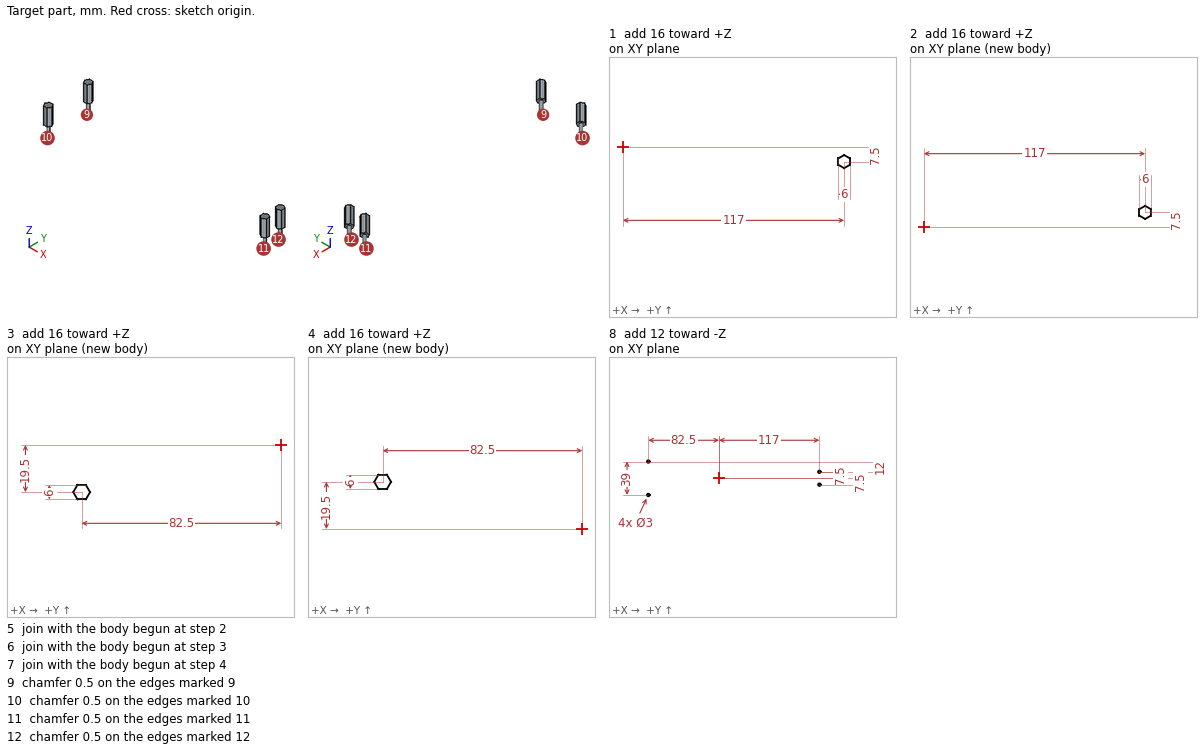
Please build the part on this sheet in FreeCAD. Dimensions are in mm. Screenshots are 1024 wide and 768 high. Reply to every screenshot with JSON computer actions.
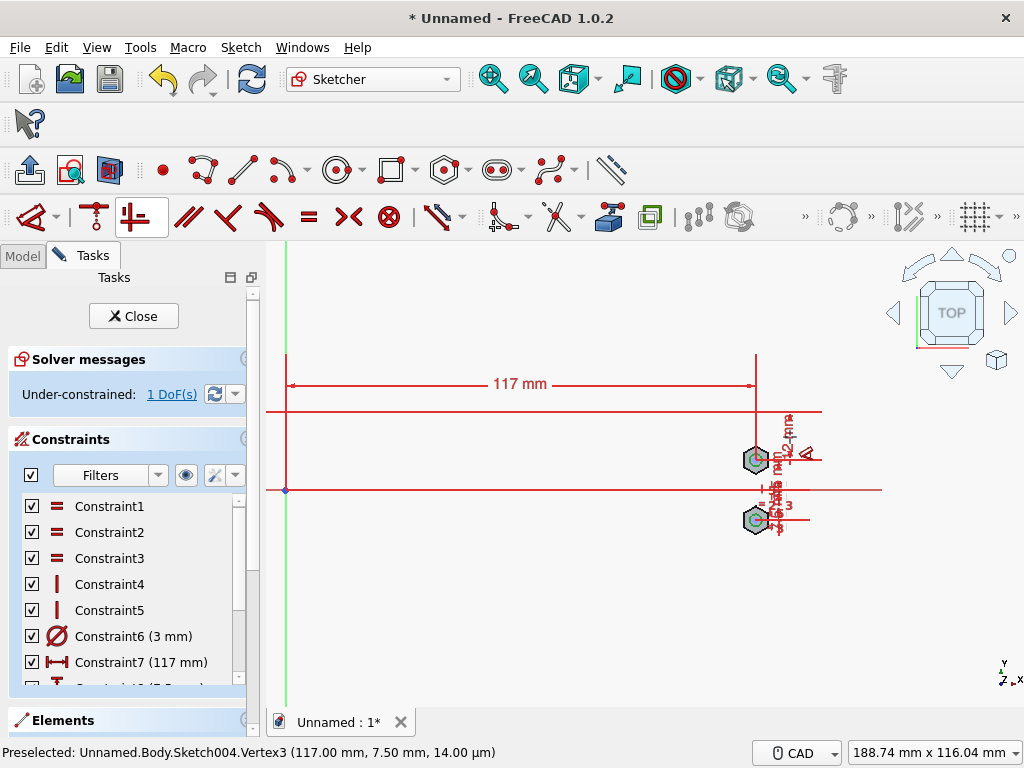
{"action": "scroll", "coordinate": [757, 461], "scroll_direction": "down", "scroll_amount": 4}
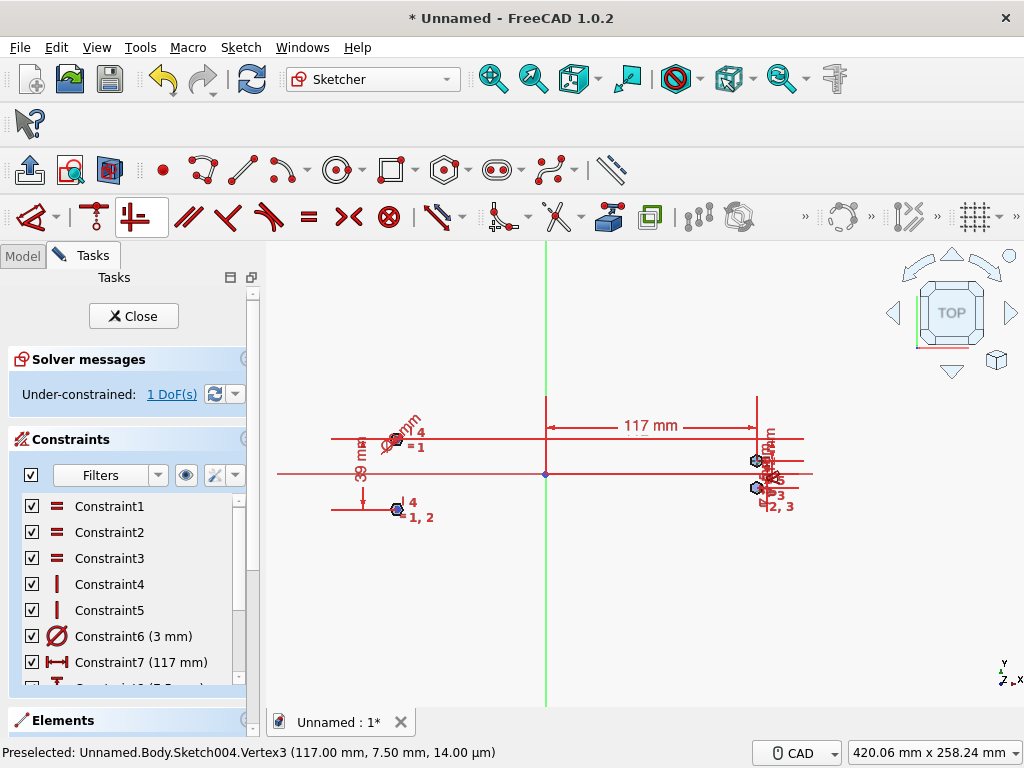
{"action": "left_click", "coordinate": [397, 439]}
{"action": "left_click", "coordinate": [471, 405]}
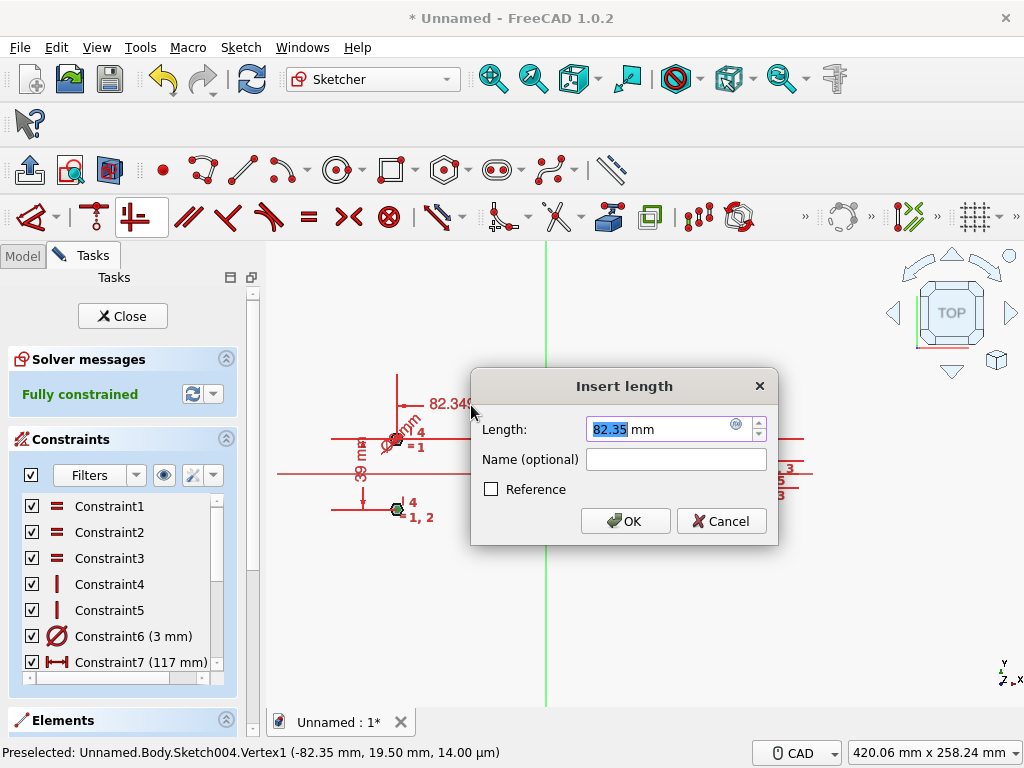
{"action": "type", "text": "82.5"}
{"action": "key", "text": "Return"}
{"action": "key", "text": "Escape"}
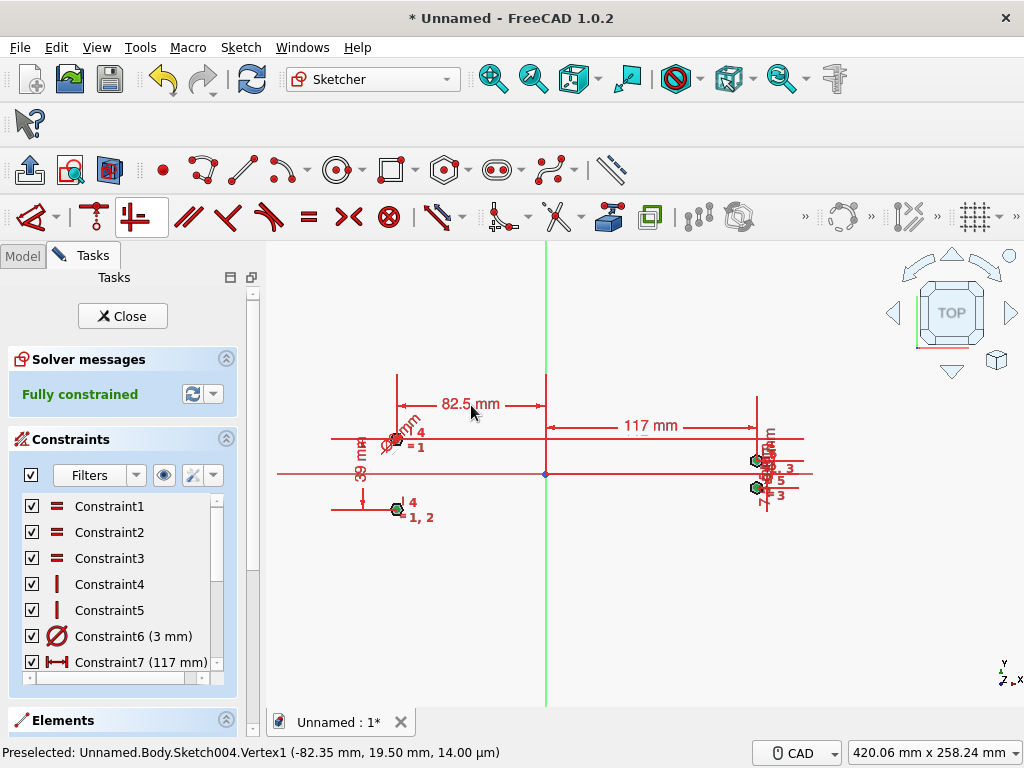
{"action": "left_click", "coordinate": [123, 316]}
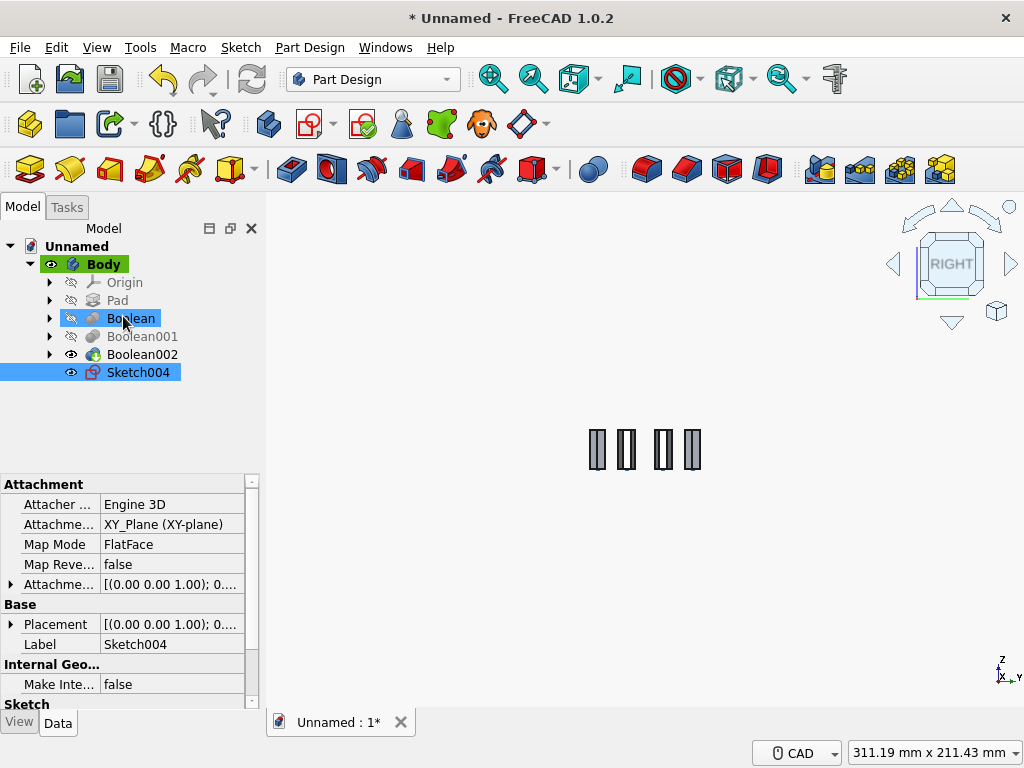
{"action": "left_click", "coordinate": [30, 170]}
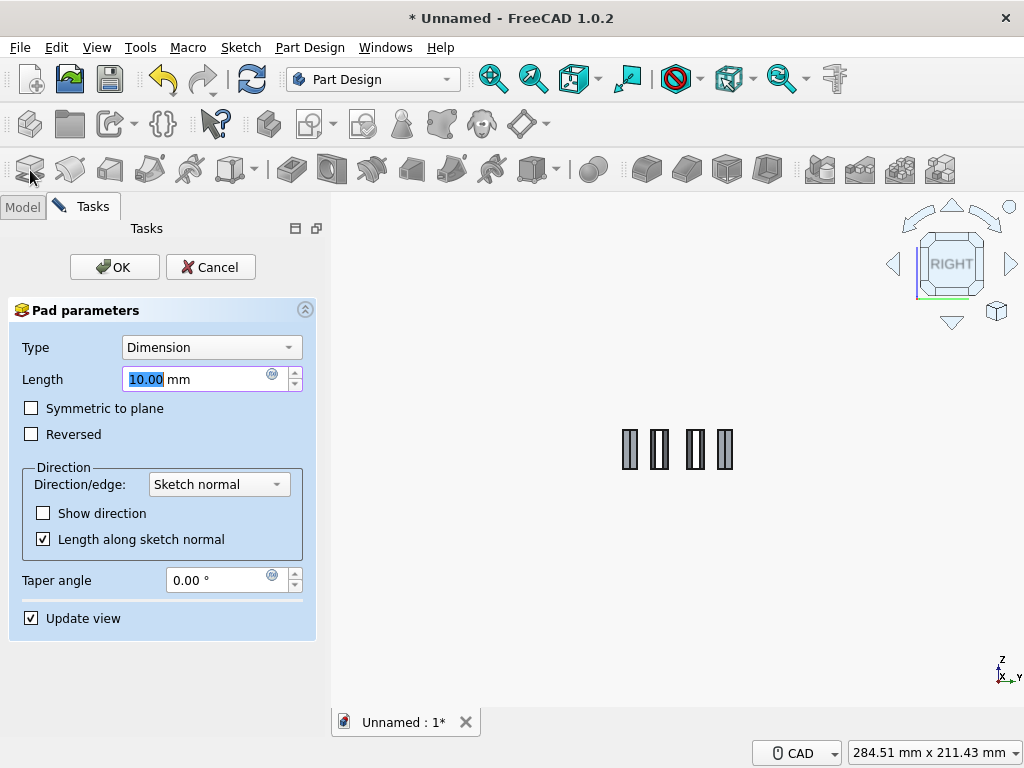
{"action": "type", "text": "12"}
{"action": "key", "text": "Tab"}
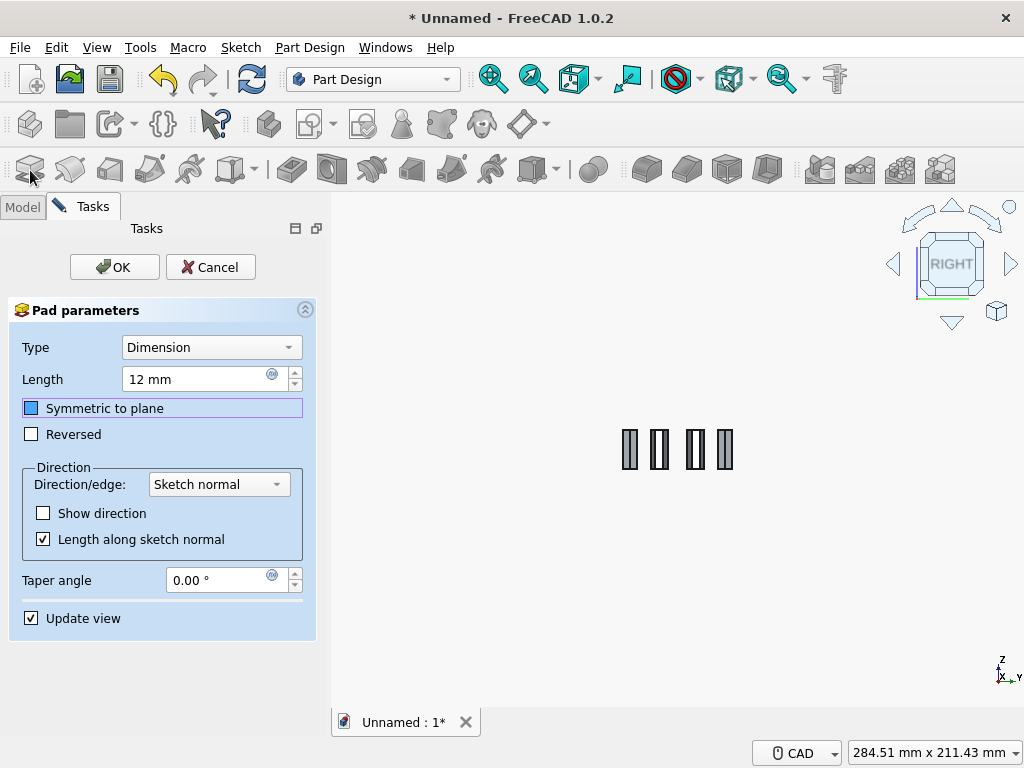
{"action": "left_click", "coordinate": [30, 434]}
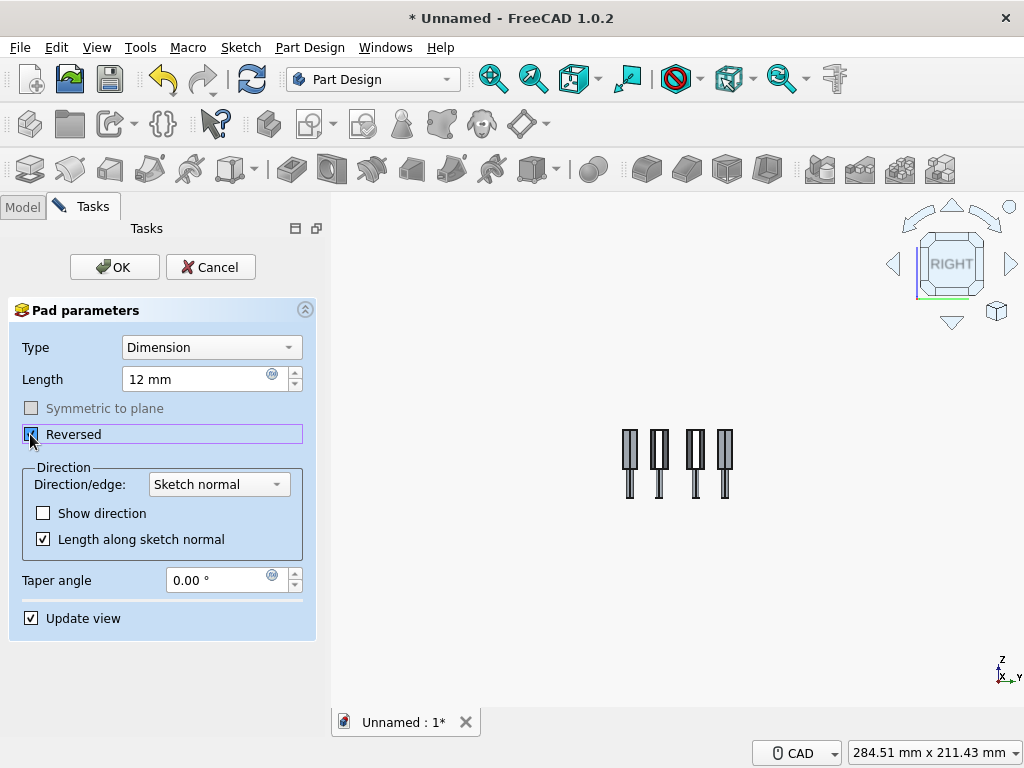
{"action": "left_click", "coordinate": [115, 267]}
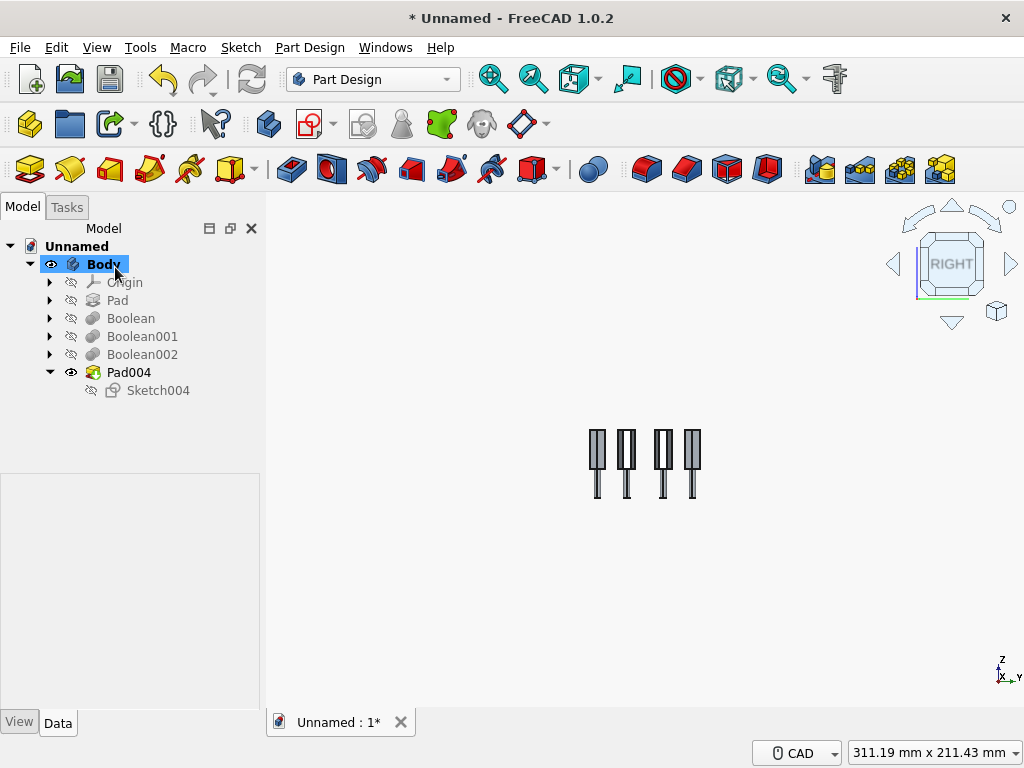
{"action": "left_click", "coordinate": [494, 80]}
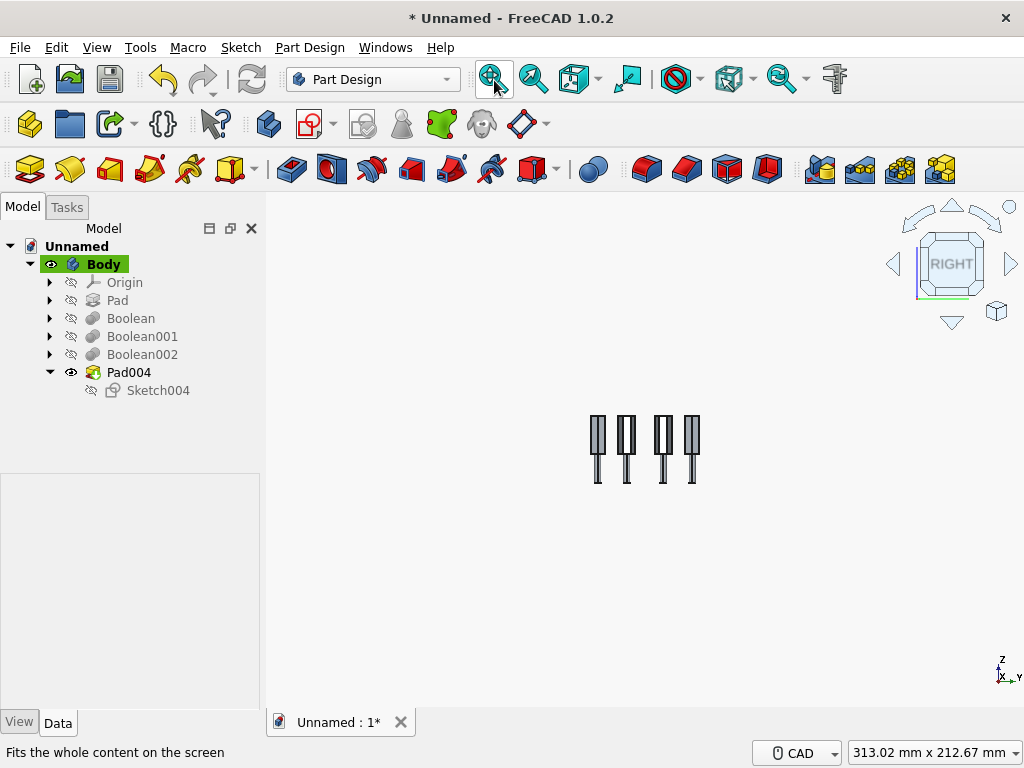
{"action": "key", "text": "0"}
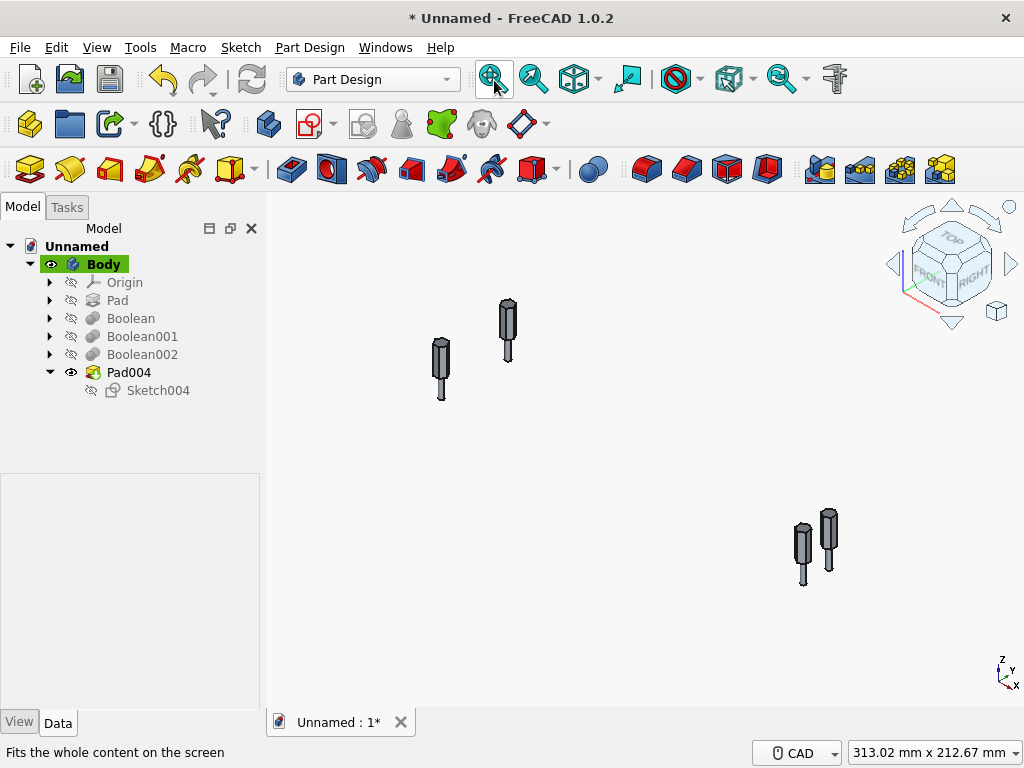
{"action": "key", "text": "2"}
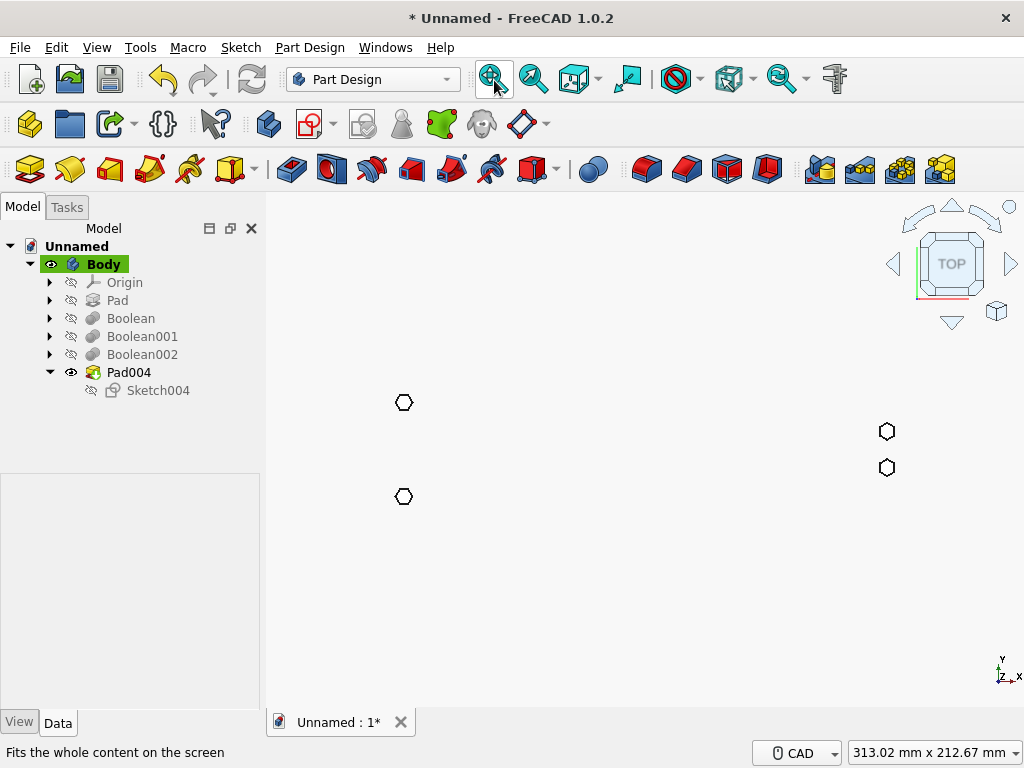
{"action": "key", "text": "1"}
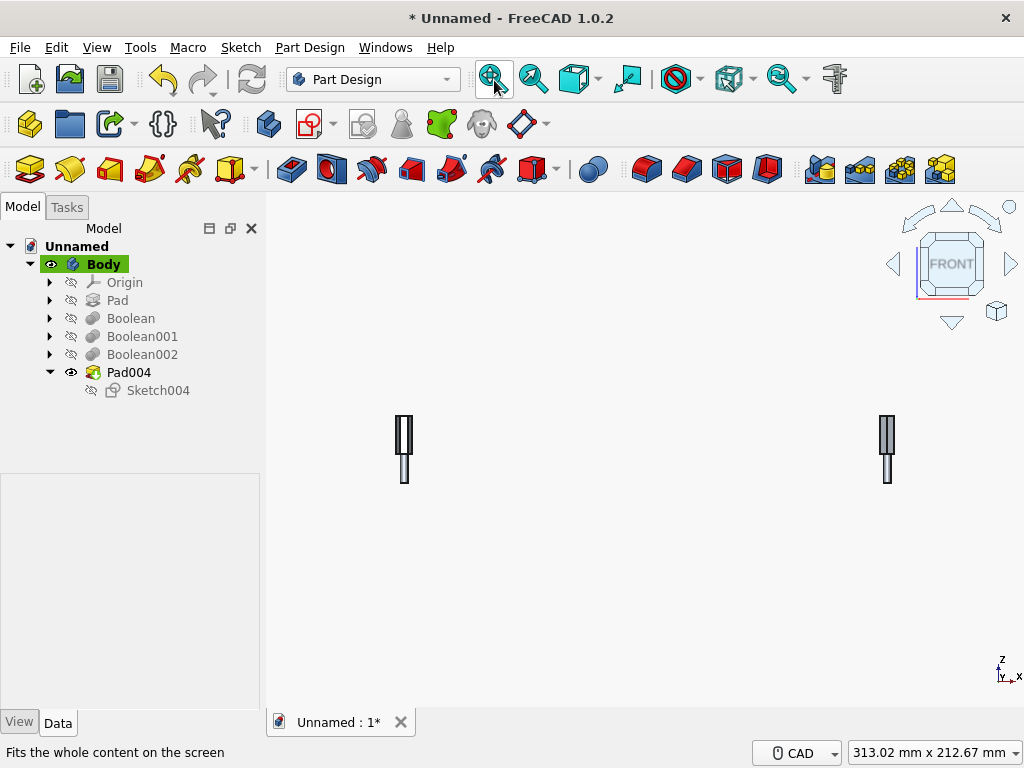
{"action": "key", "text": "3"}